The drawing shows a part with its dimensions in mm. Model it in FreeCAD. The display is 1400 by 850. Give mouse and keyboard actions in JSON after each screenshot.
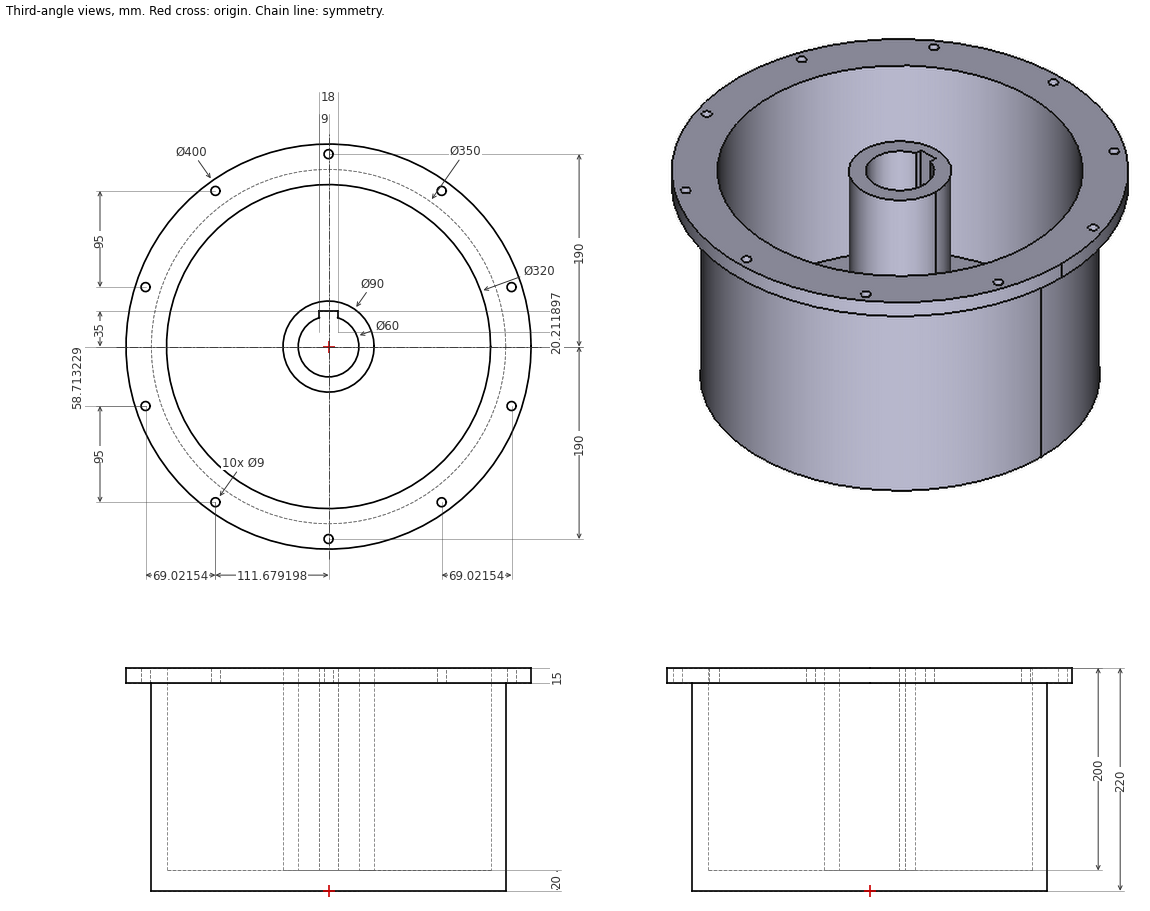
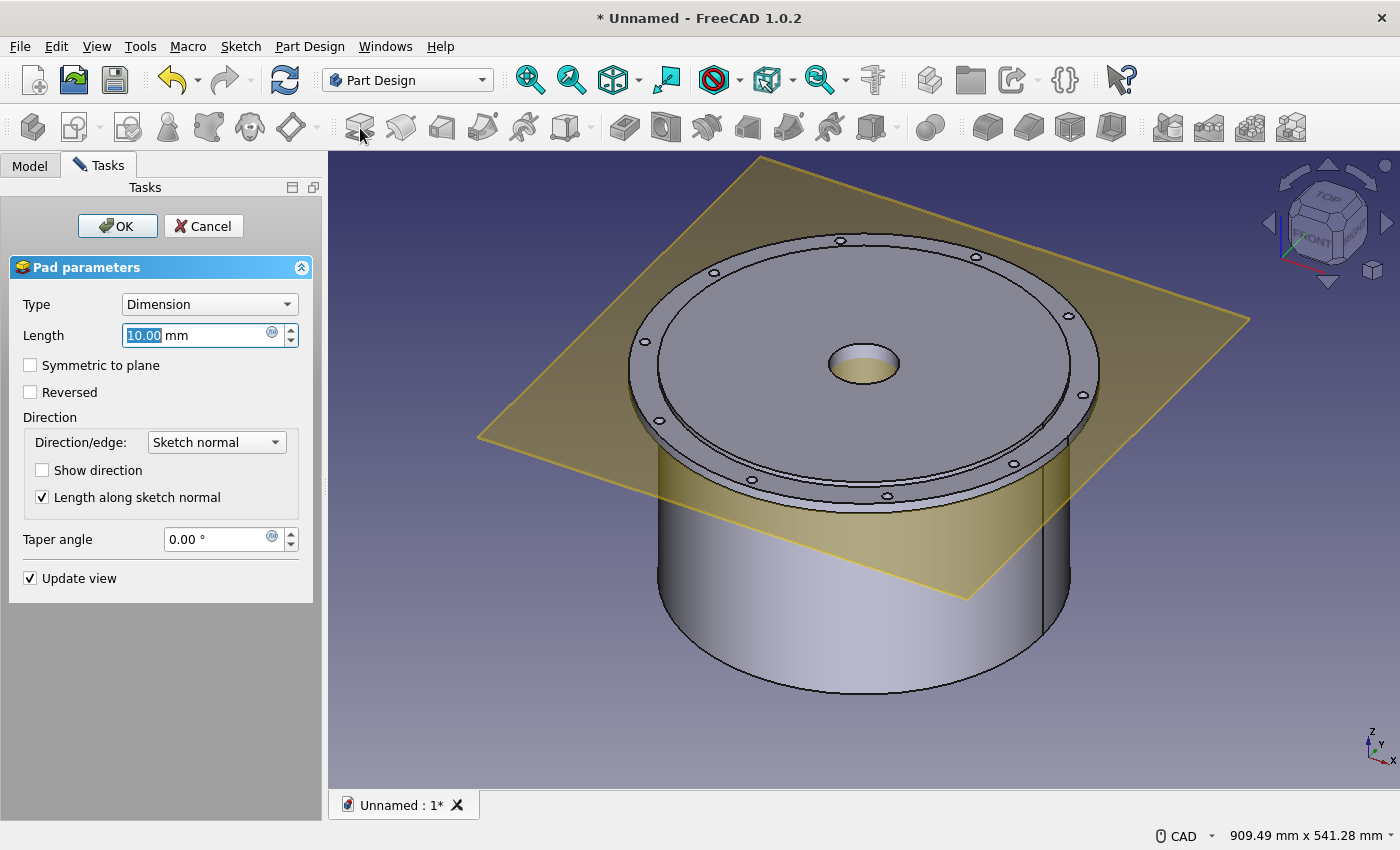
{"action": "type", "text": "15"}
{"action": "key", "text": "Tab"}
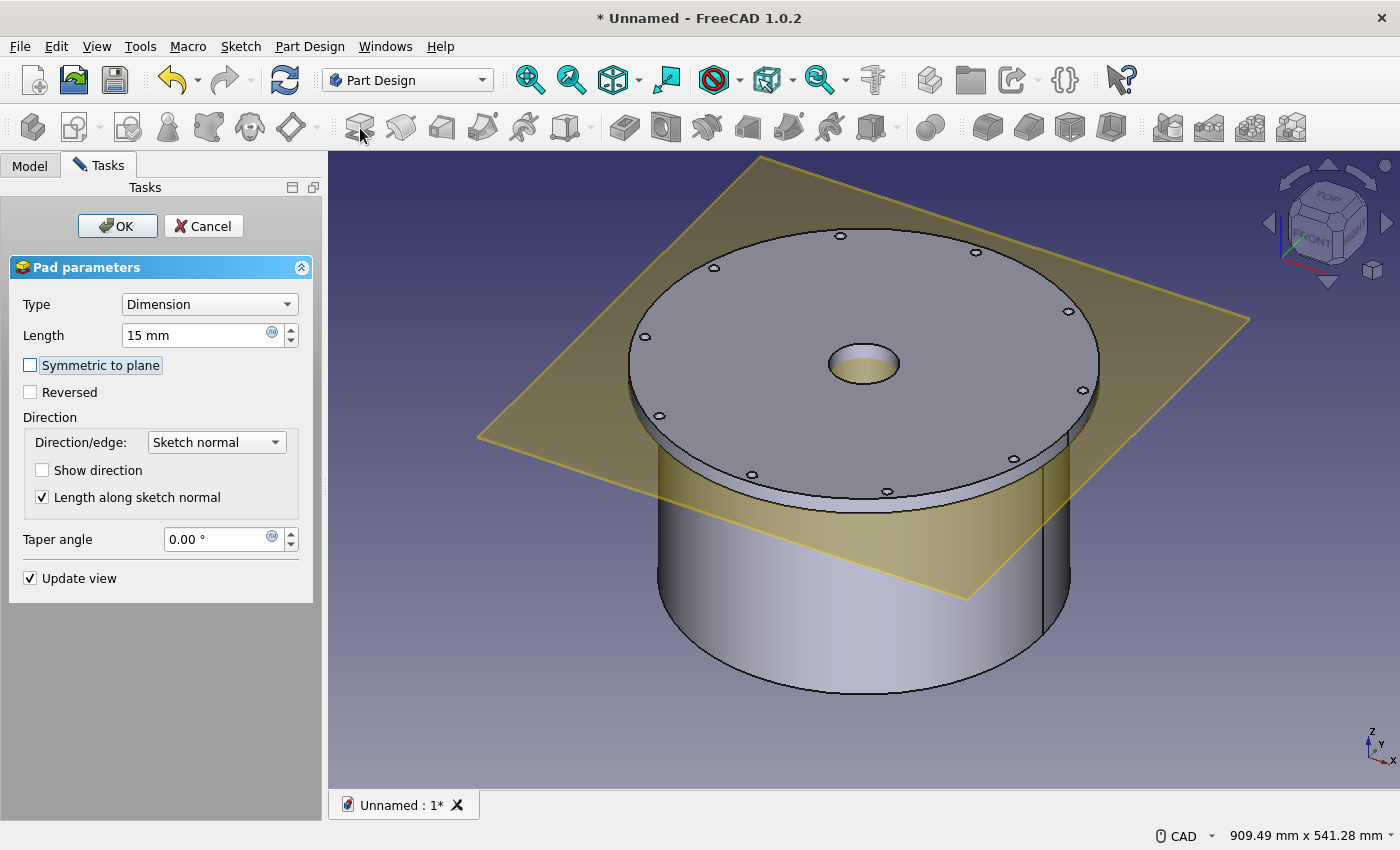
{"action": "left_click", "coordinate": [118, 226]}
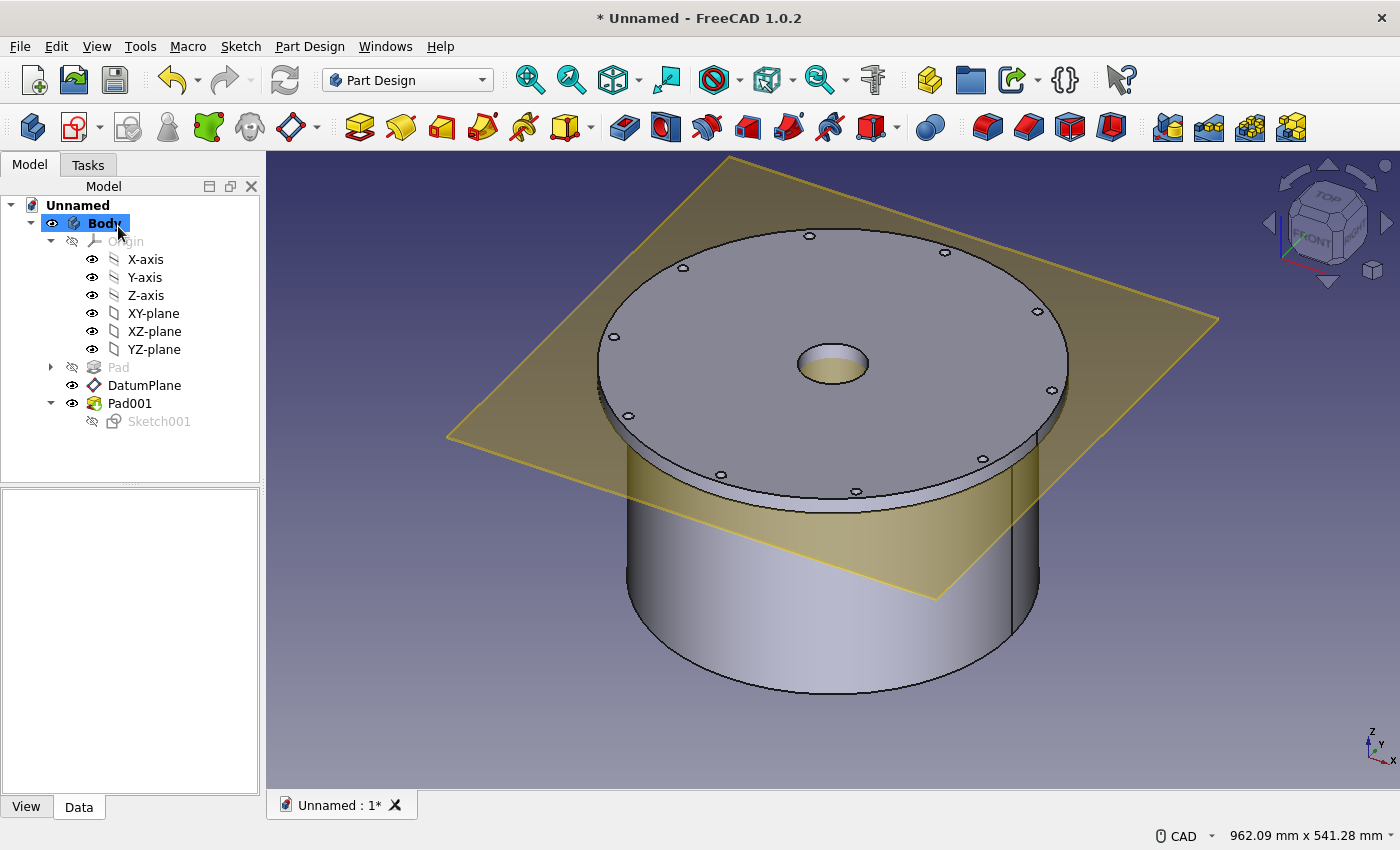
{"action": "left_click", "coordinate": [117, 385]}
{"action": "key", "text": "space"}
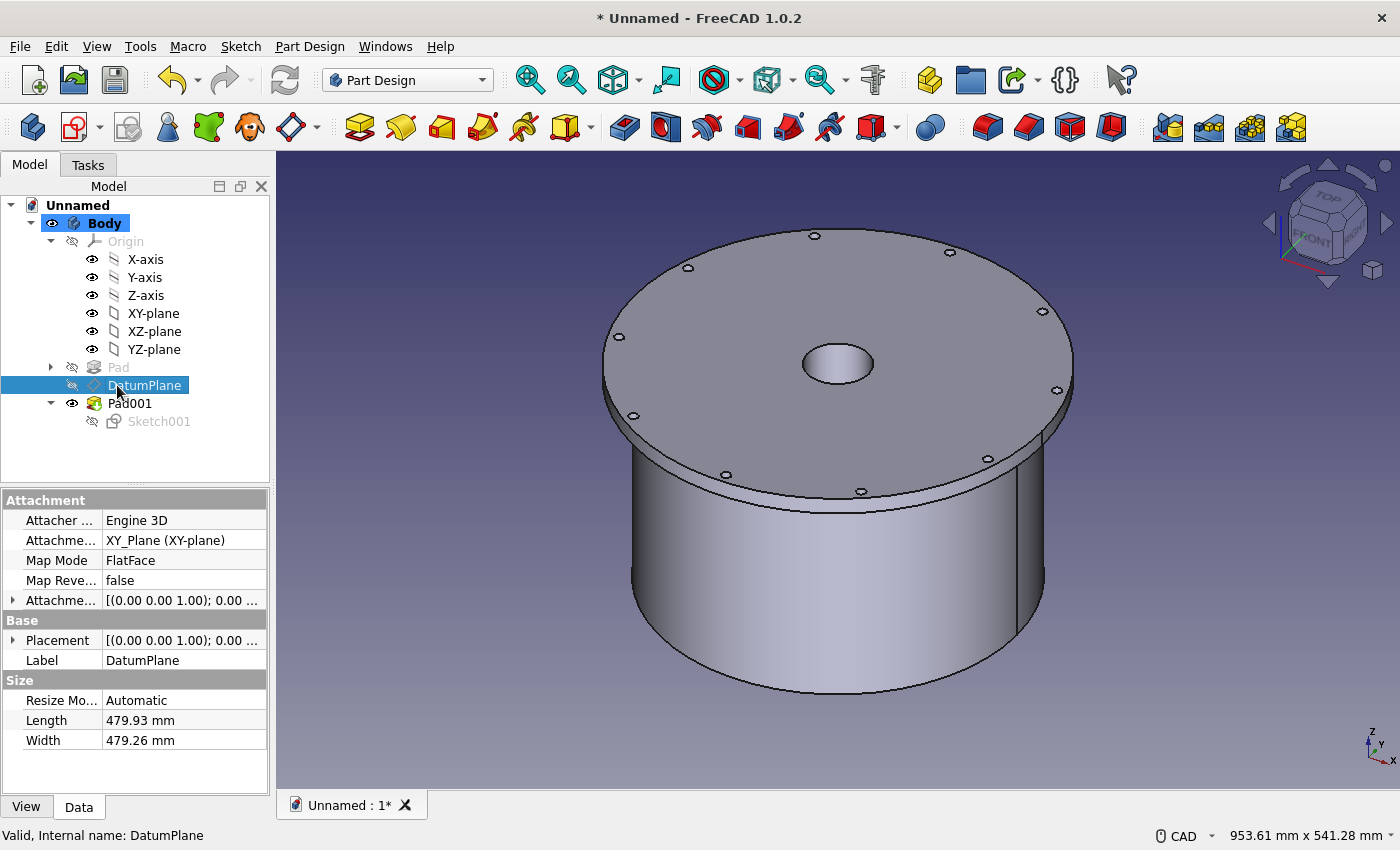
{"action": "left_click", "coordinate": [955, 401]}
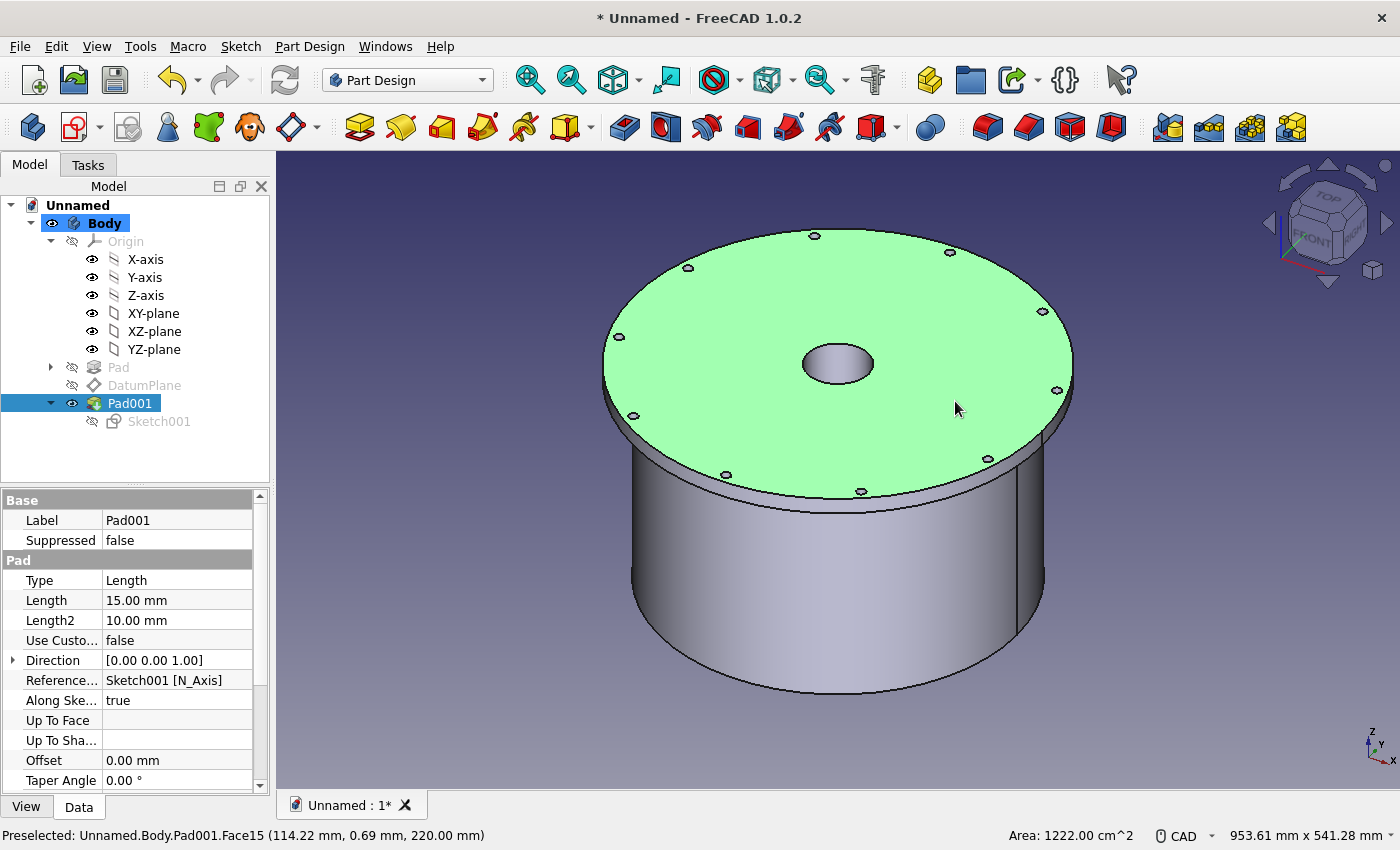
{"action": "left_click", "coordinate": [74, 128]}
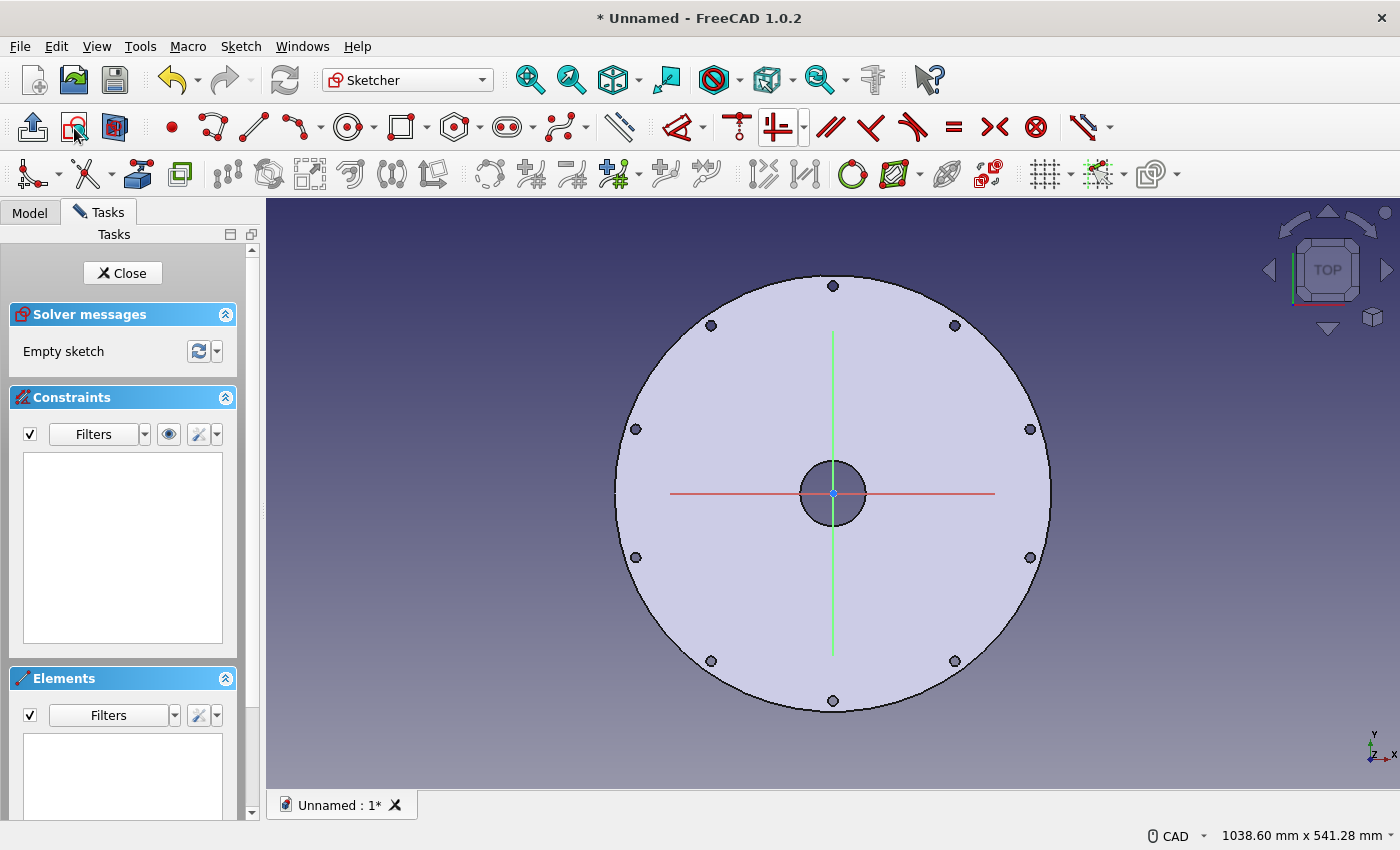
{"action": "left_click", "coordinate": [348, 128]}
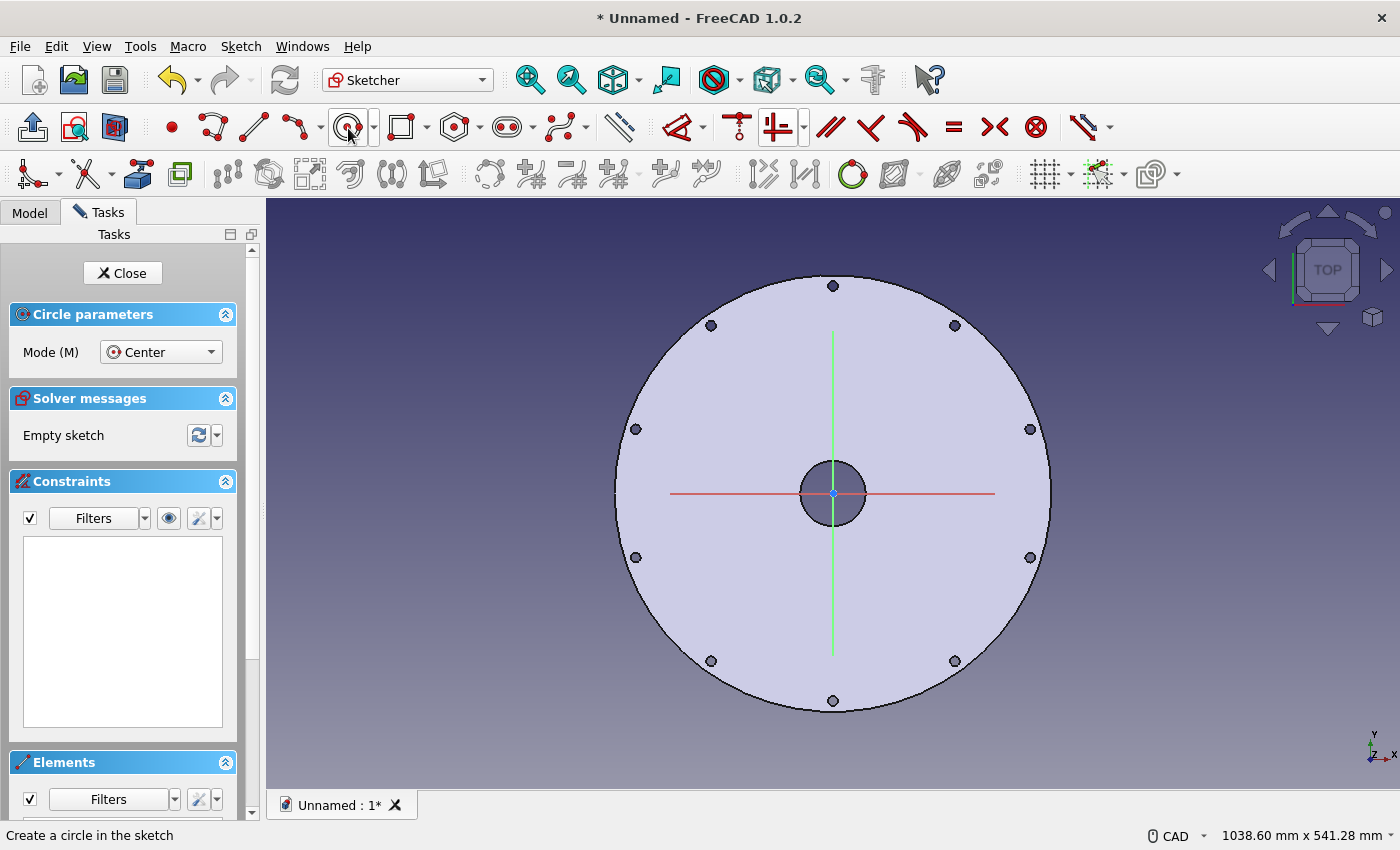
{"action": "left_click", "coordinate": [833, 494]}
{"action": "mouse_move", "coordinate": [957, 370]}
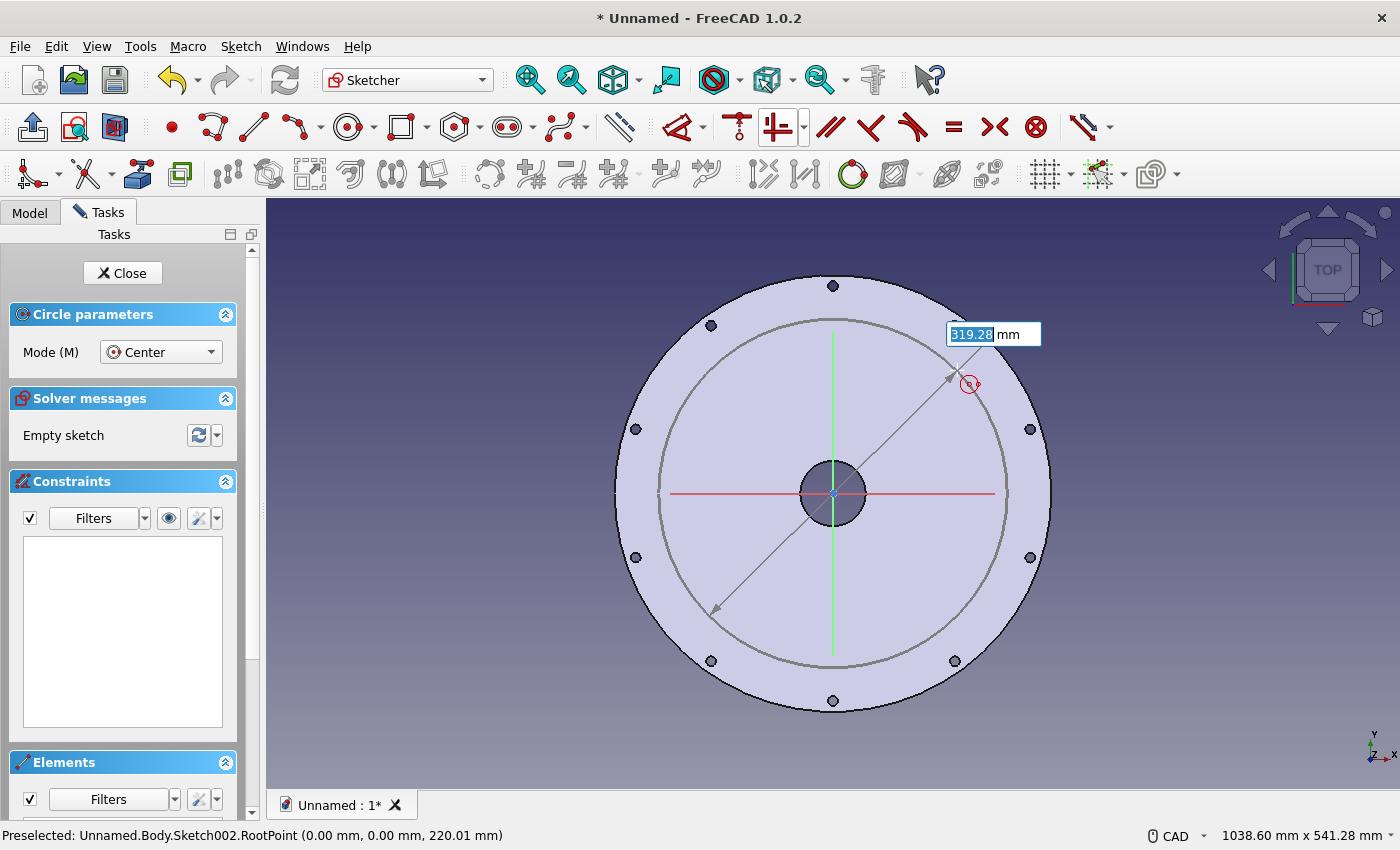
{"action": "type", "text": "320"}
{"action": "key", "text": "Return"}